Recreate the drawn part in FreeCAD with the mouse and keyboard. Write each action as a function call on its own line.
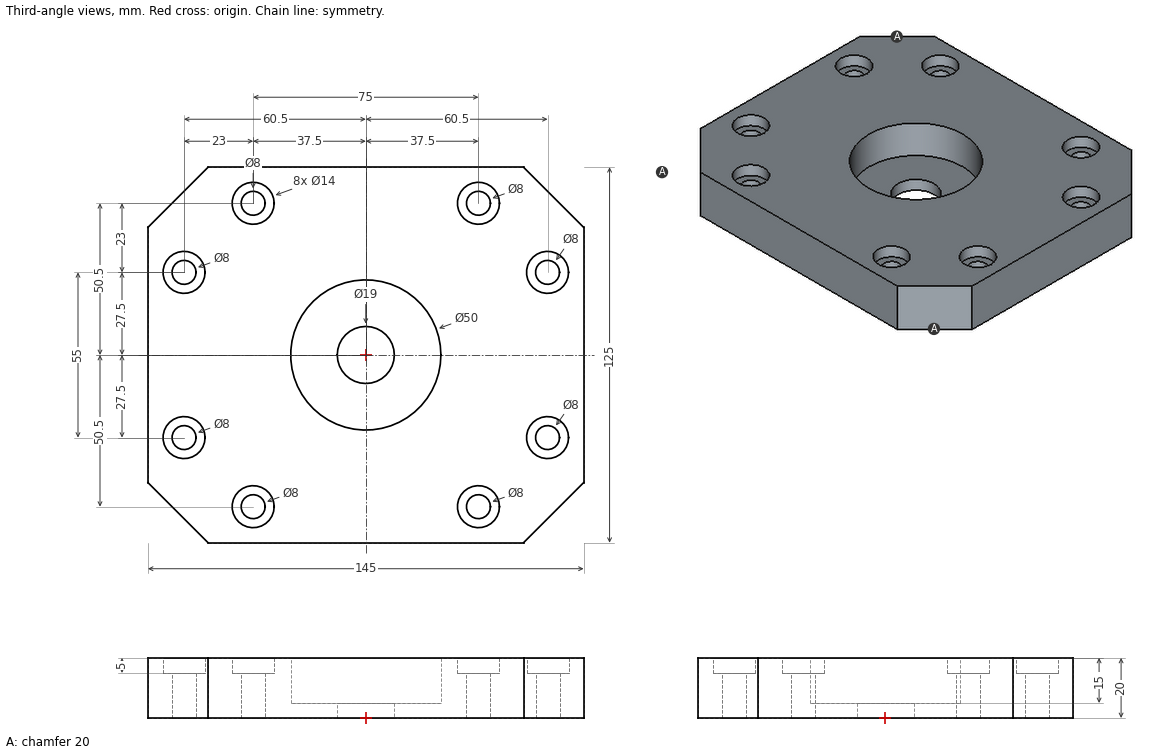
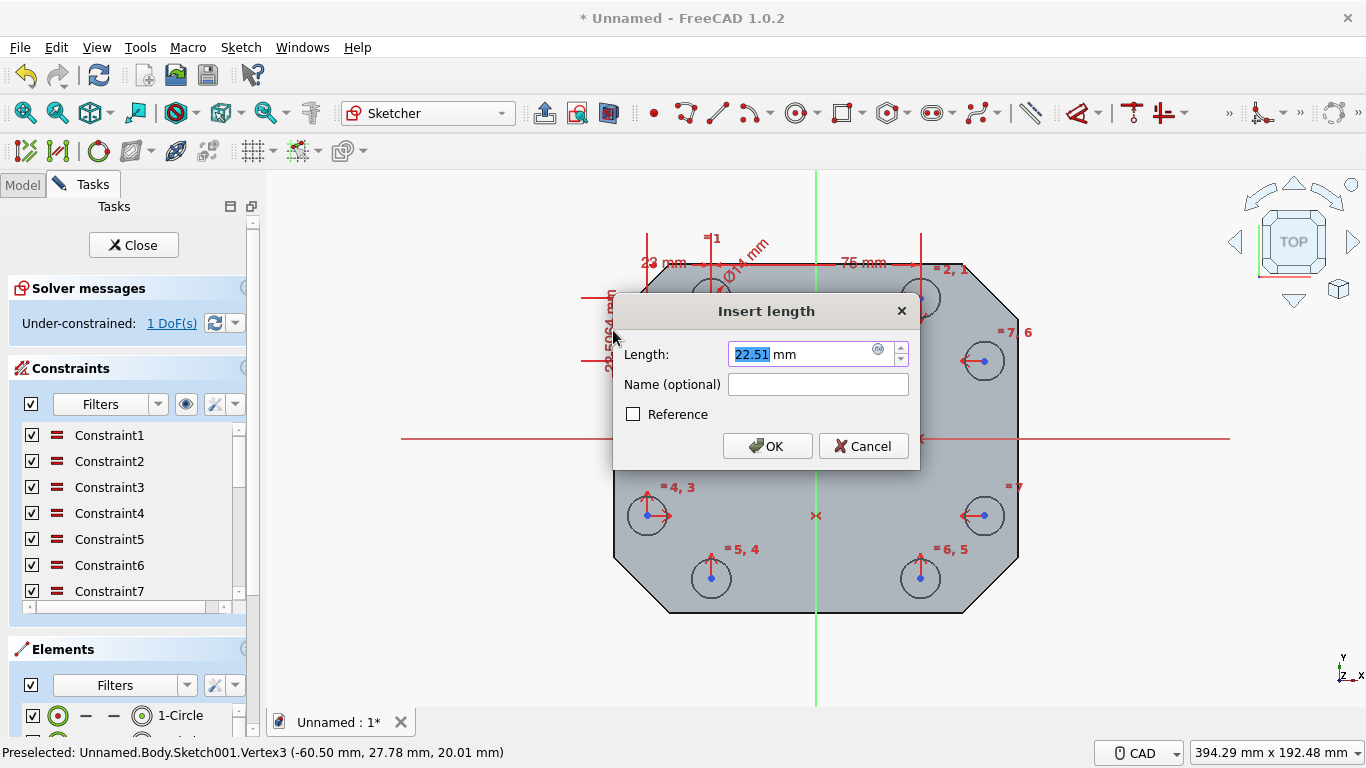
text(23)
key(Return)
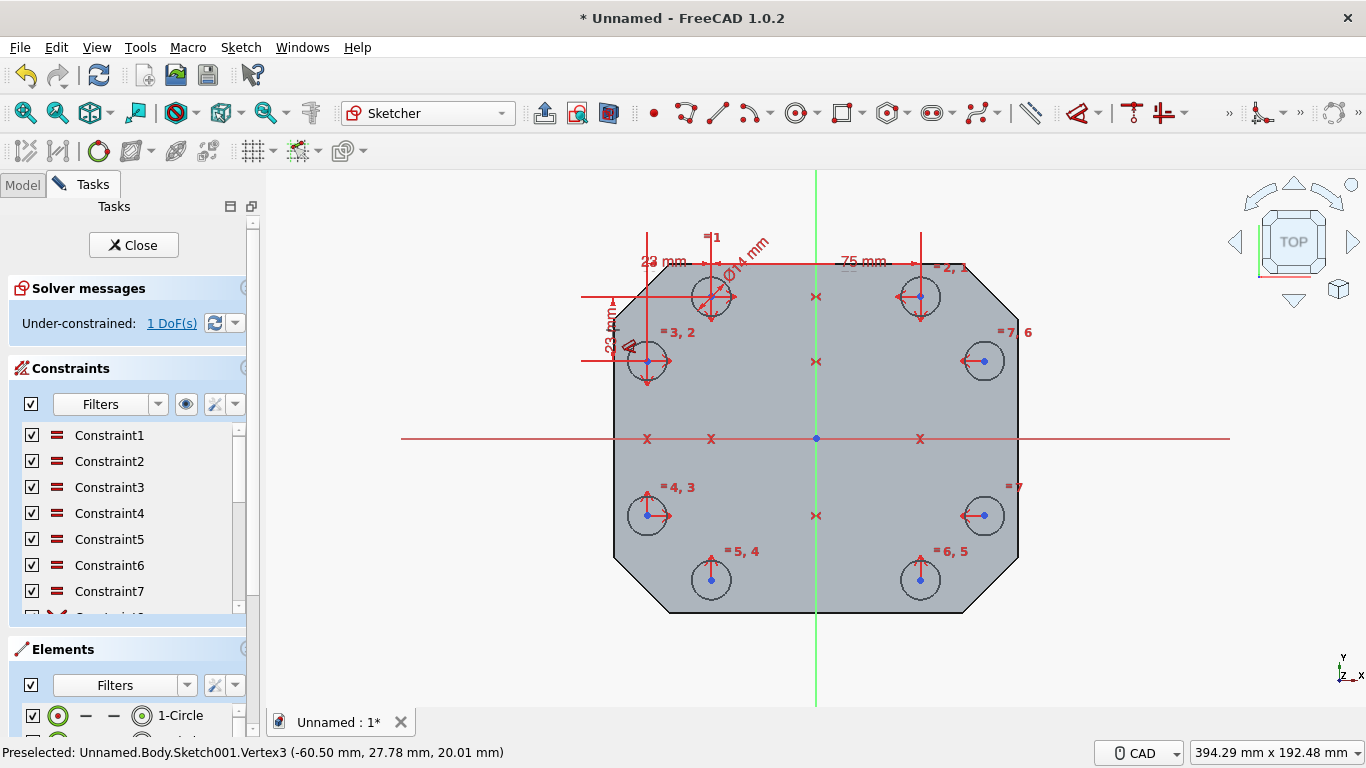
click(647, 361)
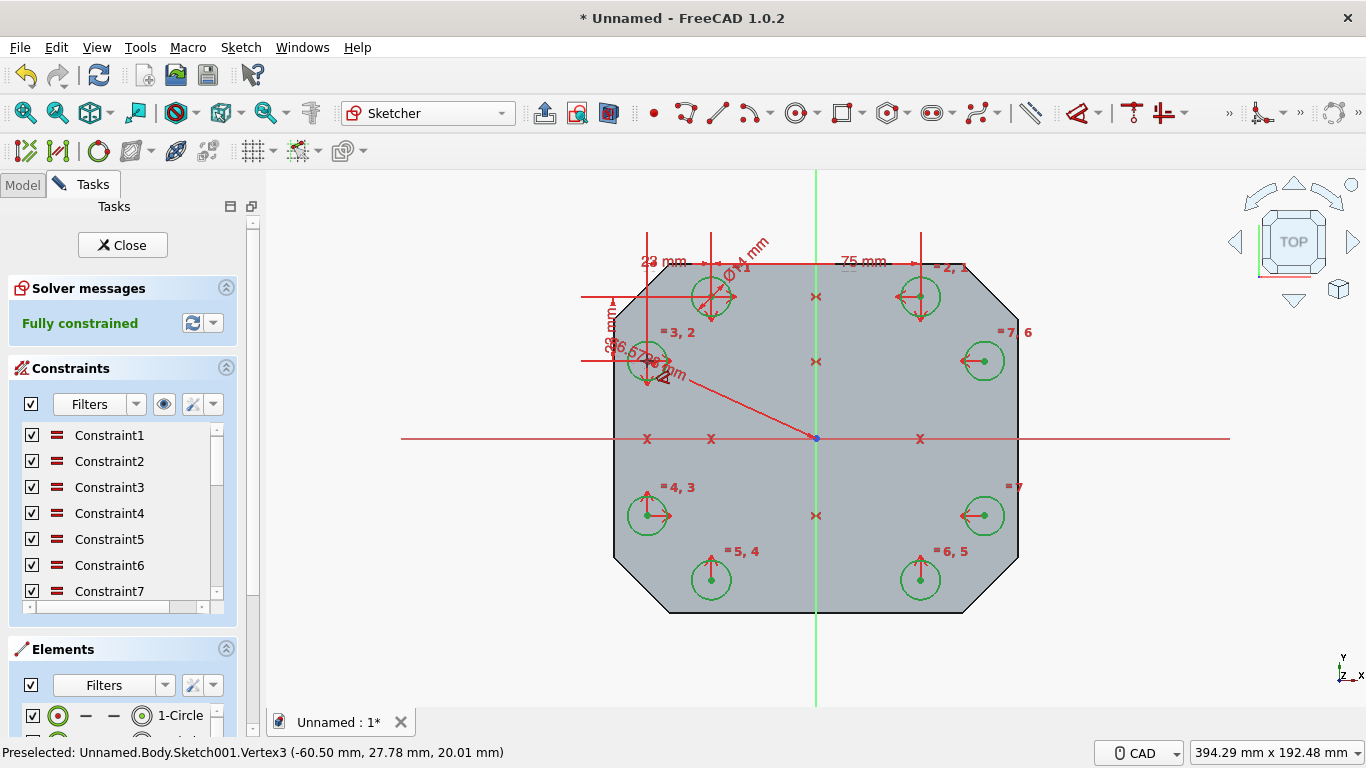
click(647, 516)
click(613, 403)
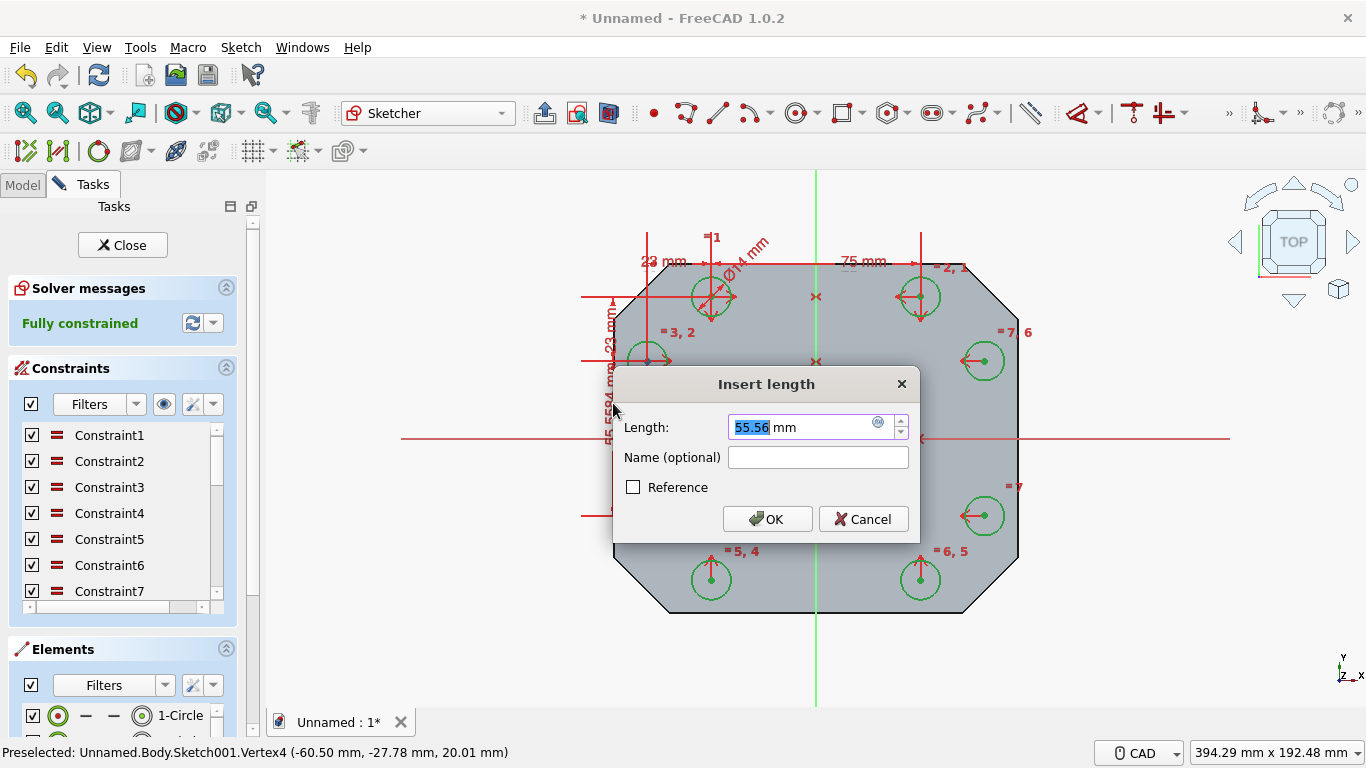
text(55)
key(Return)
key(Escape)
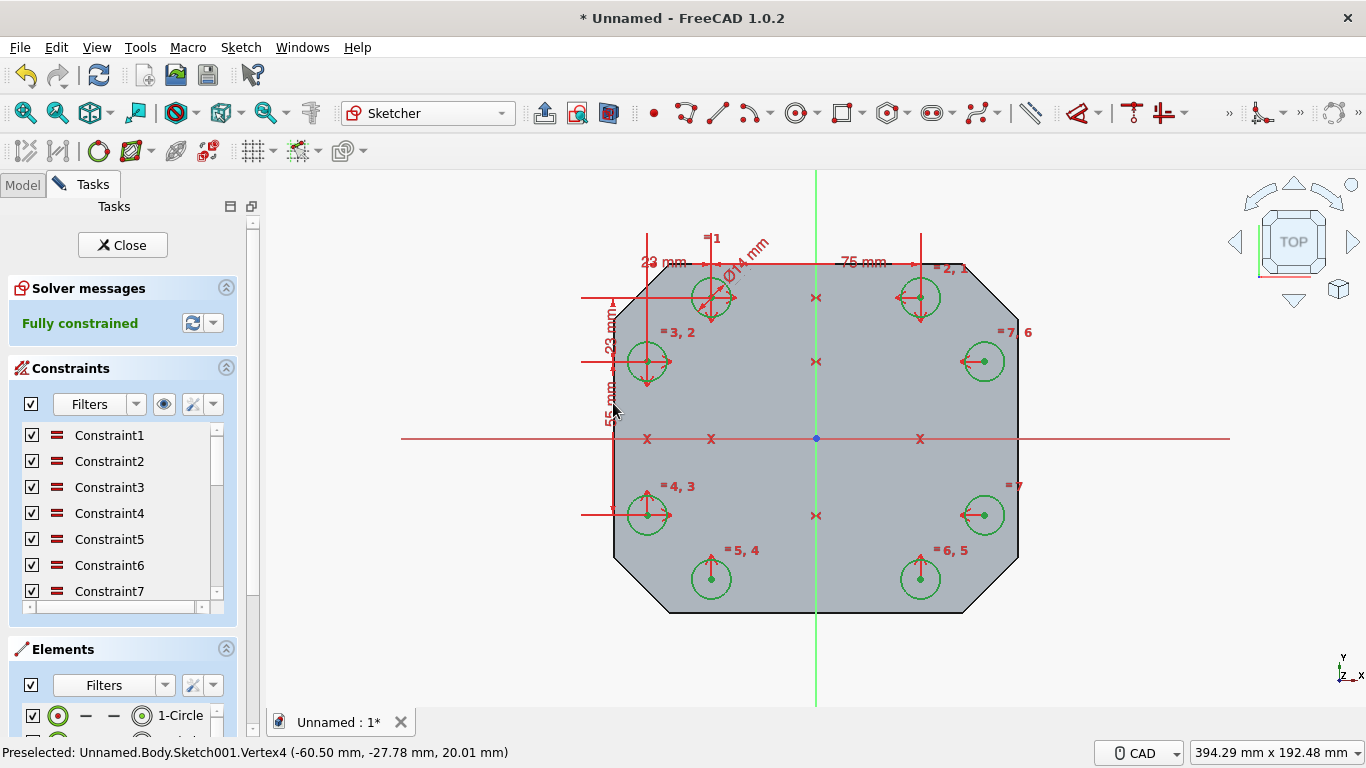
click(123, 245)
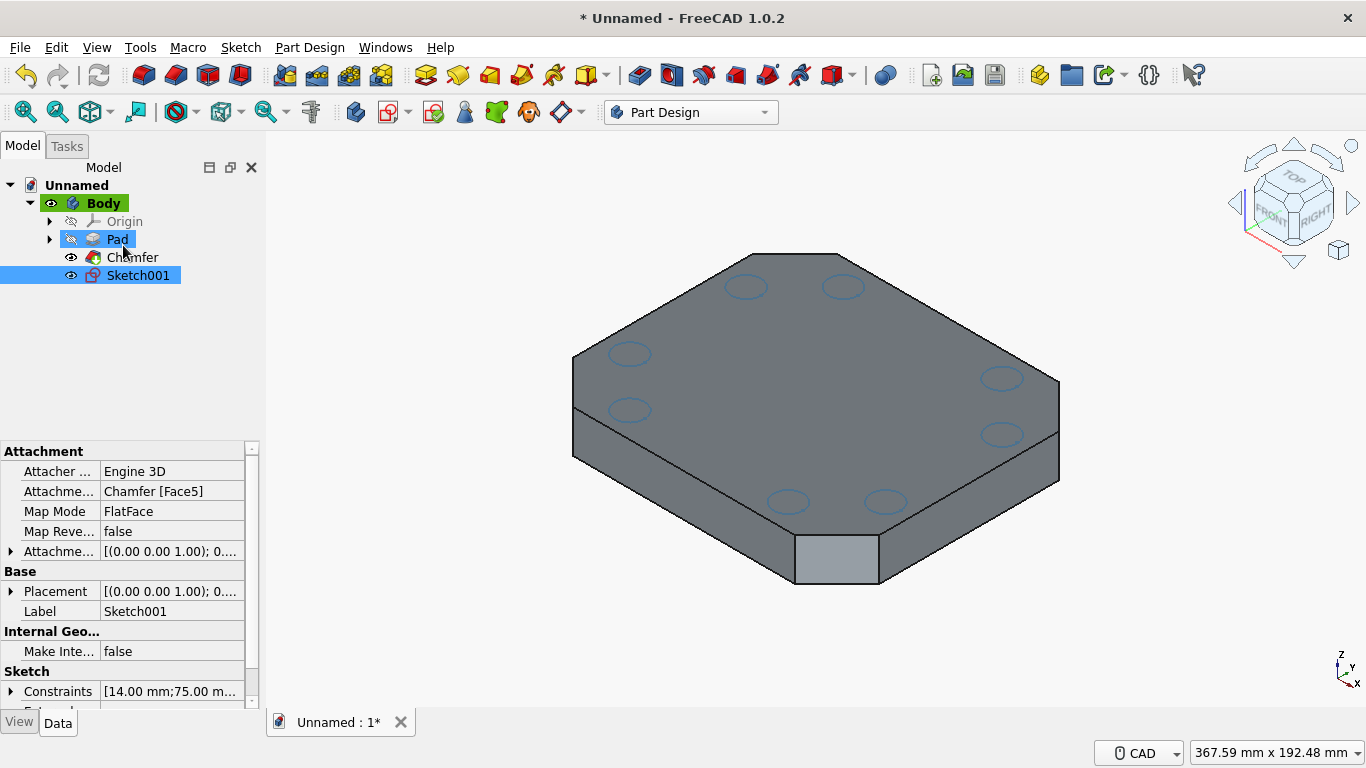
click(640, 76)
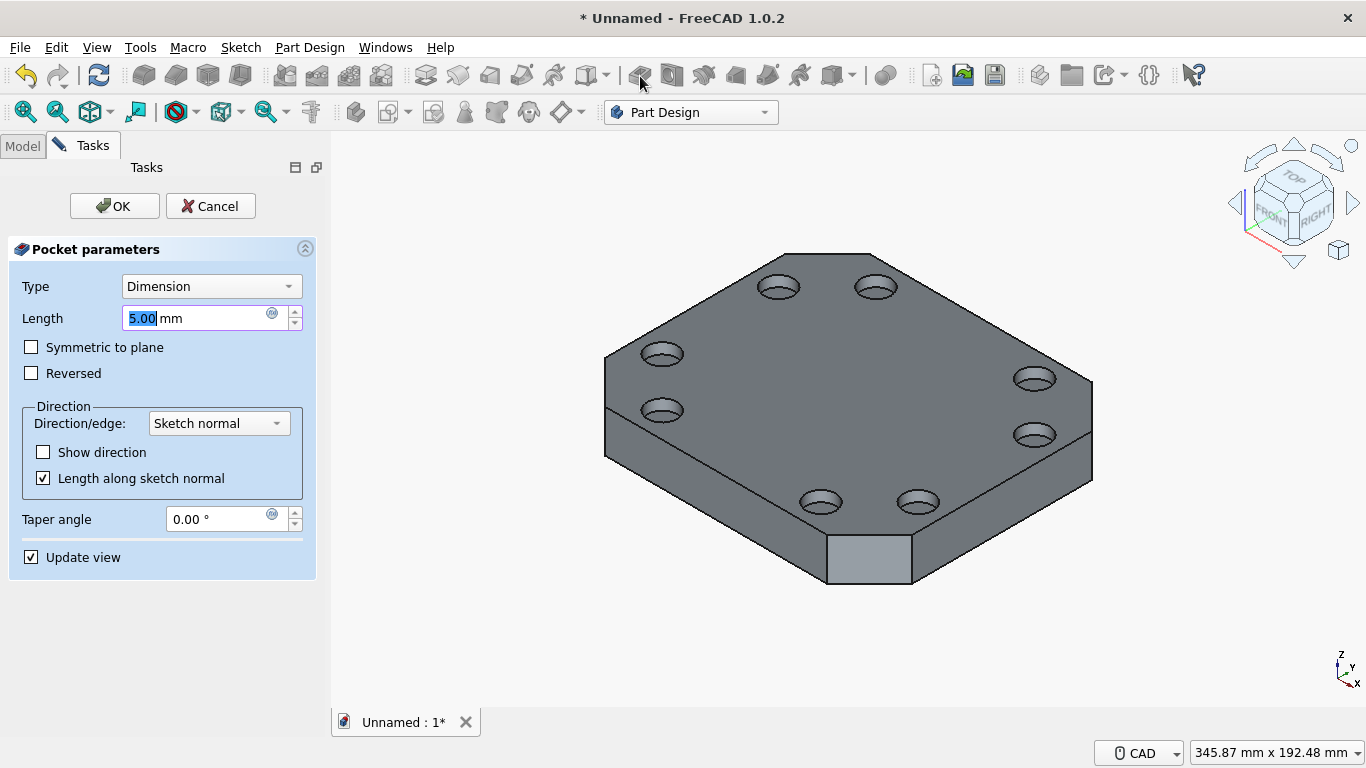
text(5)
key(Tab)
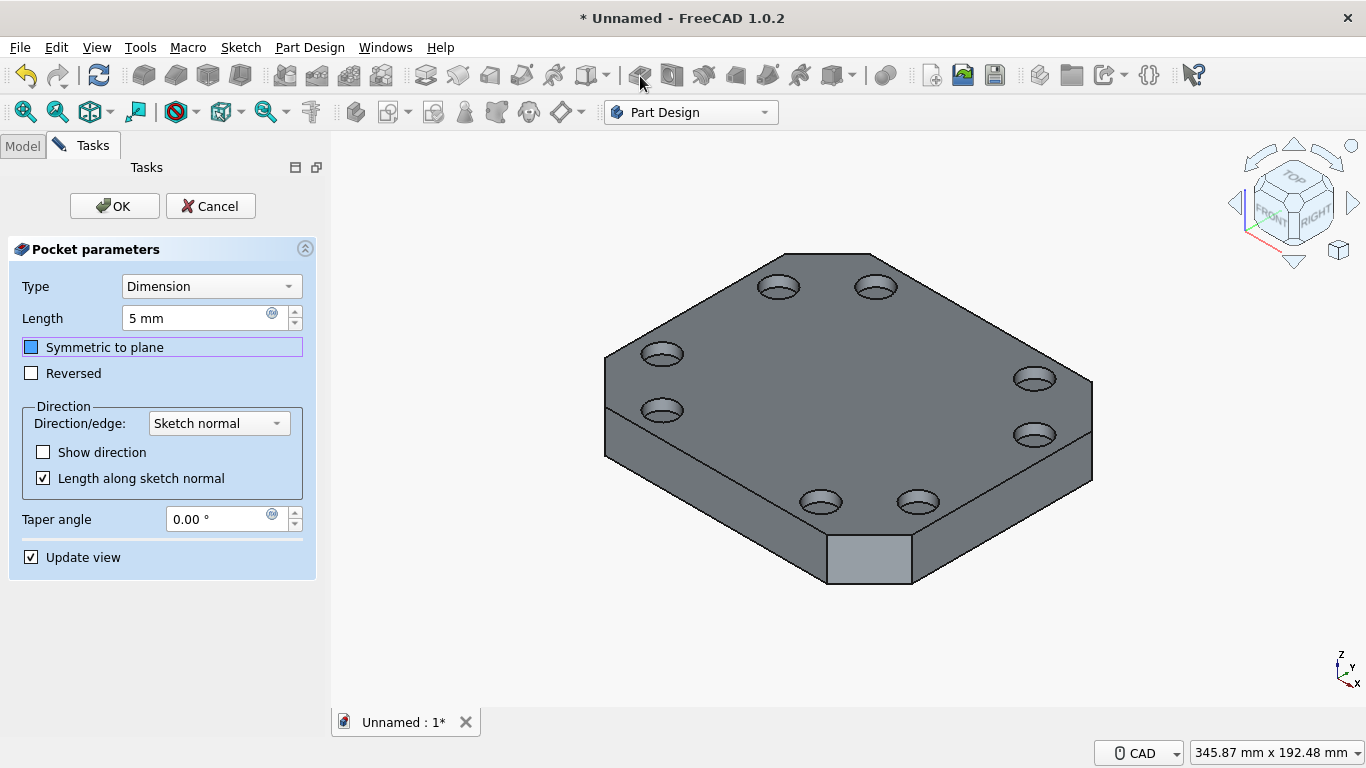
click(115, 206)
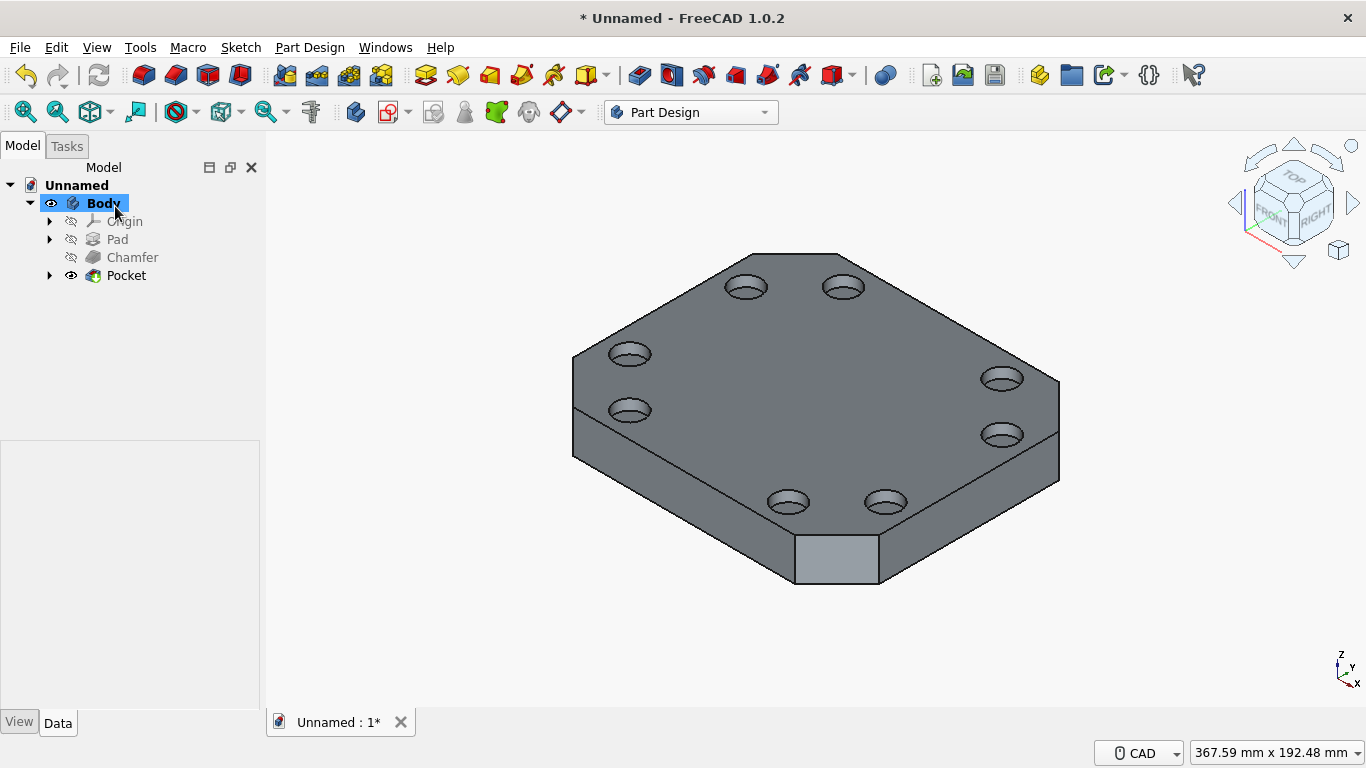
key(2)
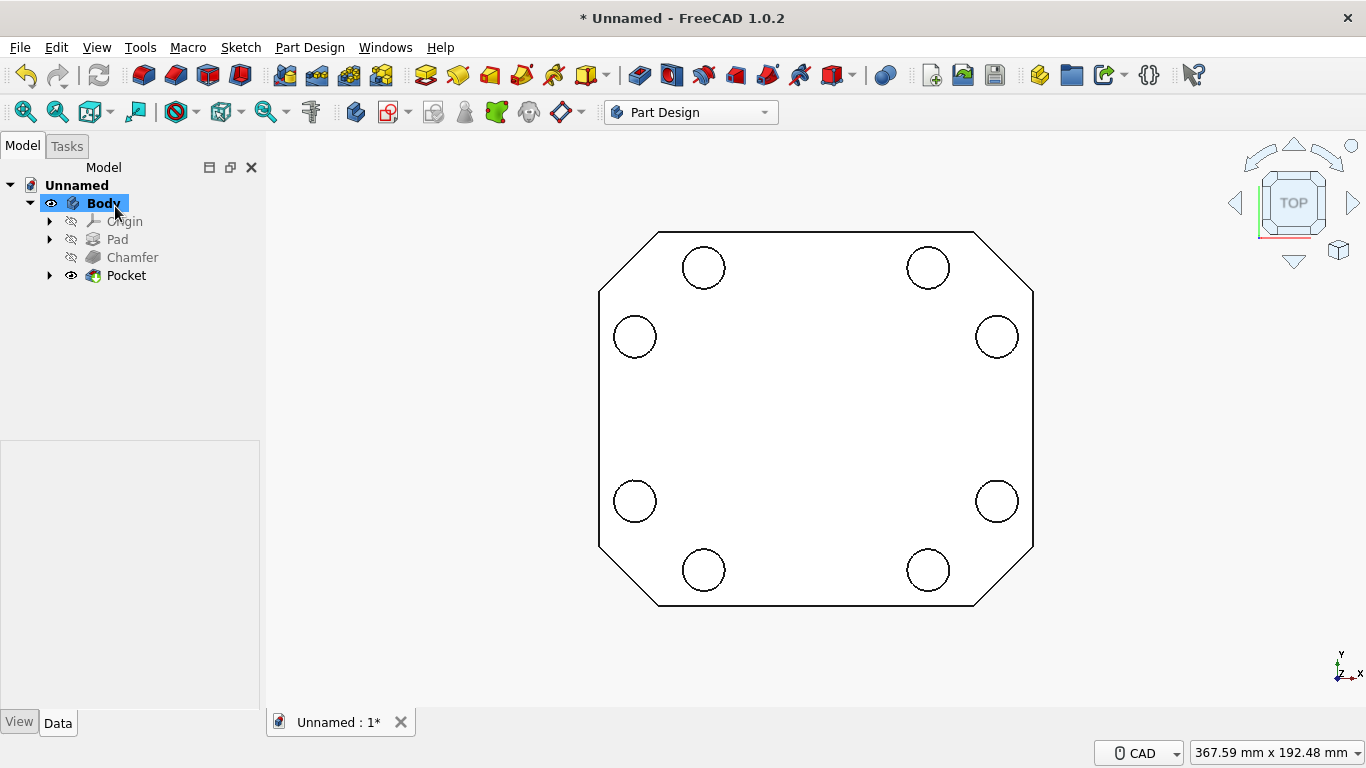
click(635, 336)